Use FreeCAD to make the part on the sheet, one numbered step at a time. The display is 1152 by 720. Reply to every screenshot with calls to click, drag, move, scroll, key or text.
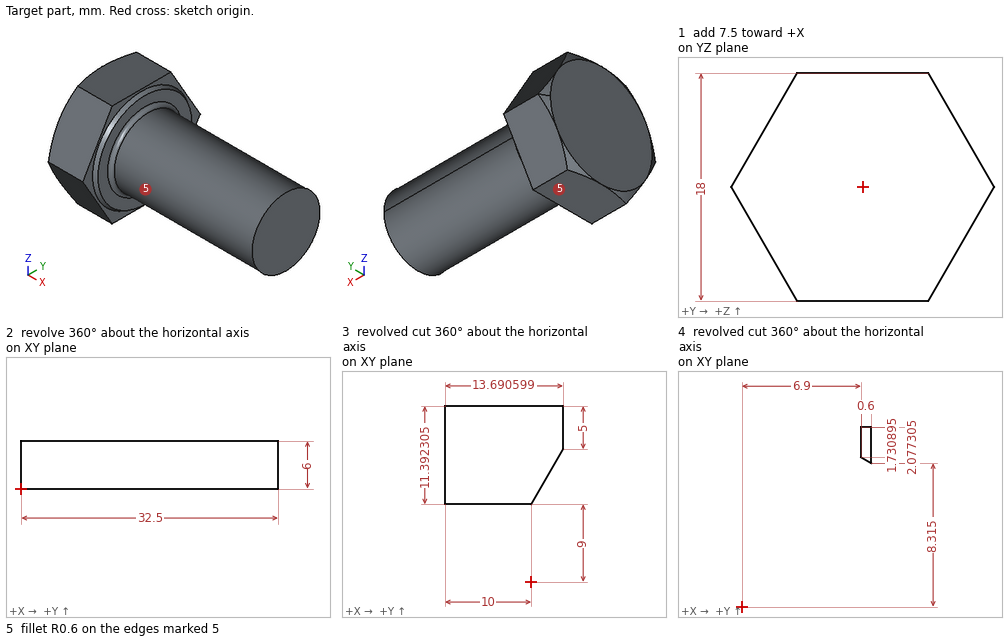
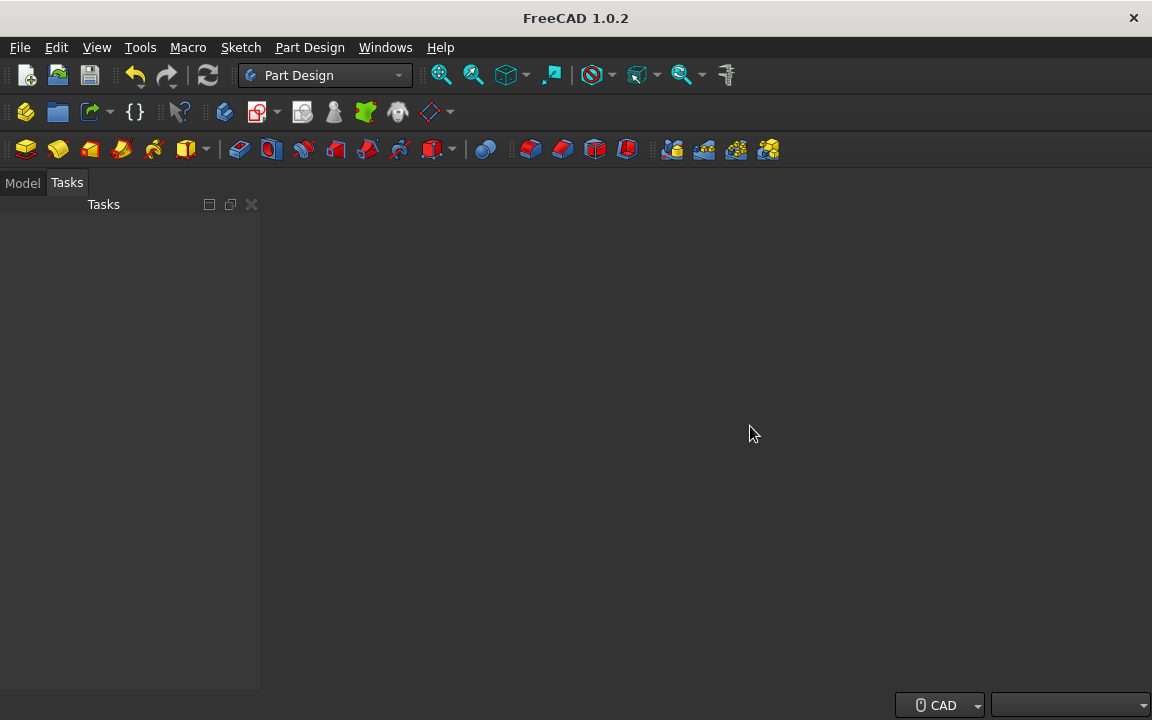
click(26, 76)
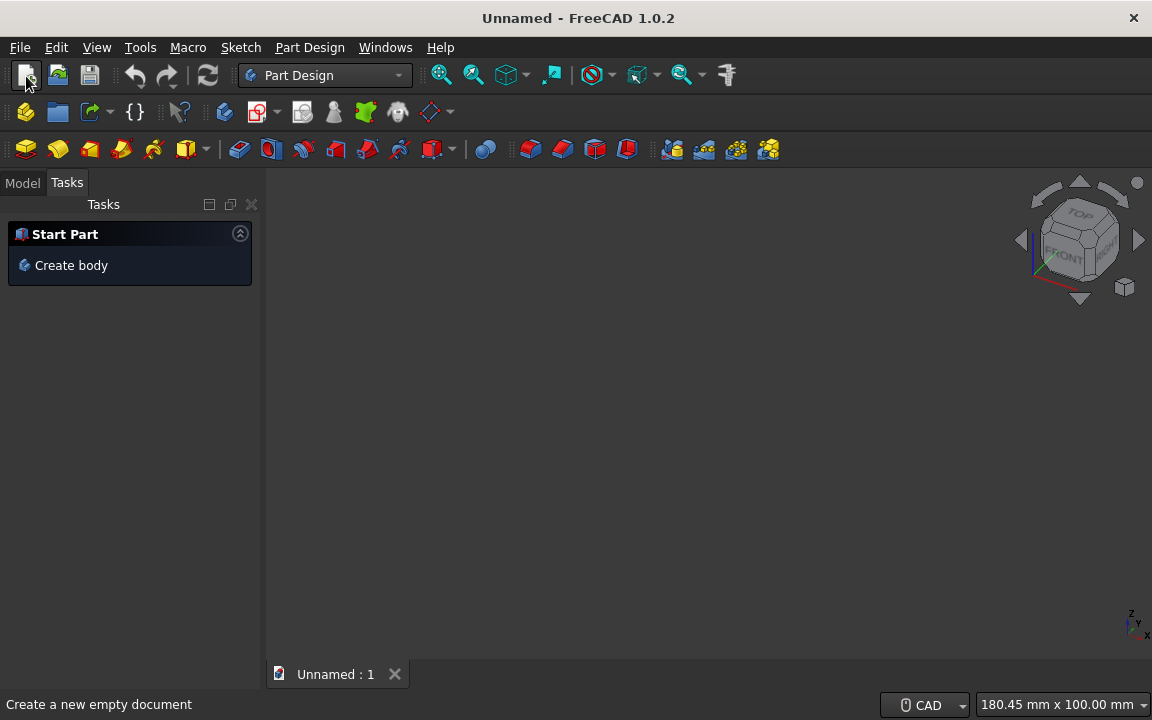
click(258, 112)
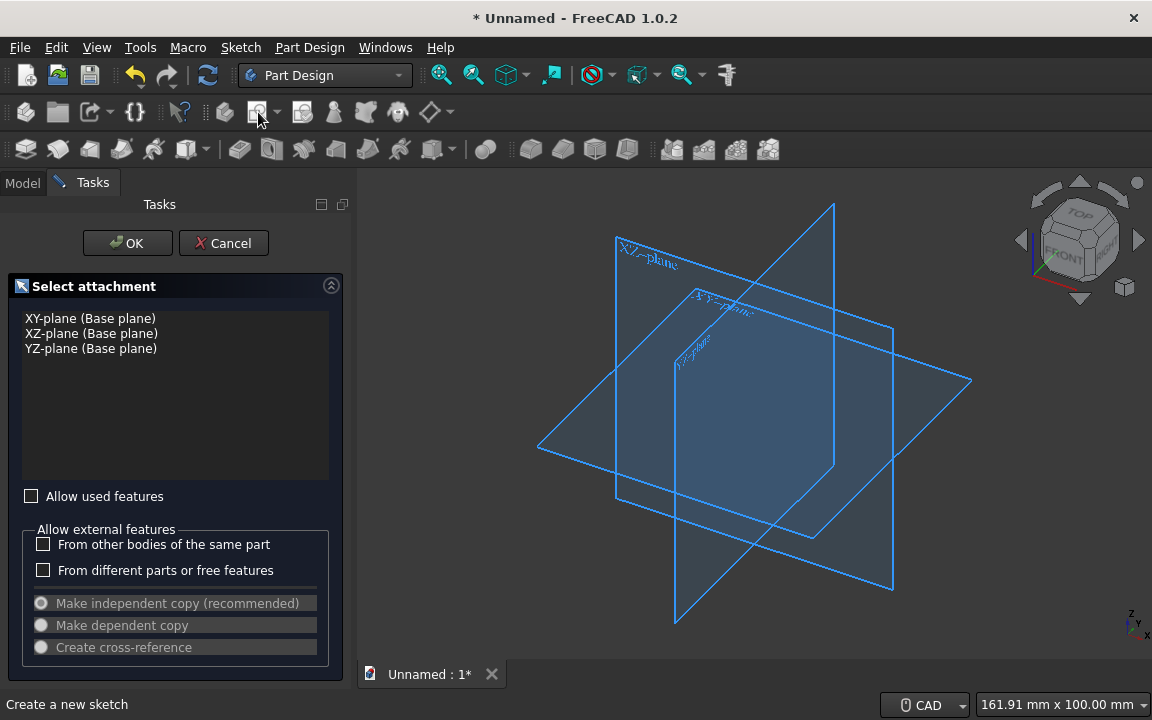
click(82, 348)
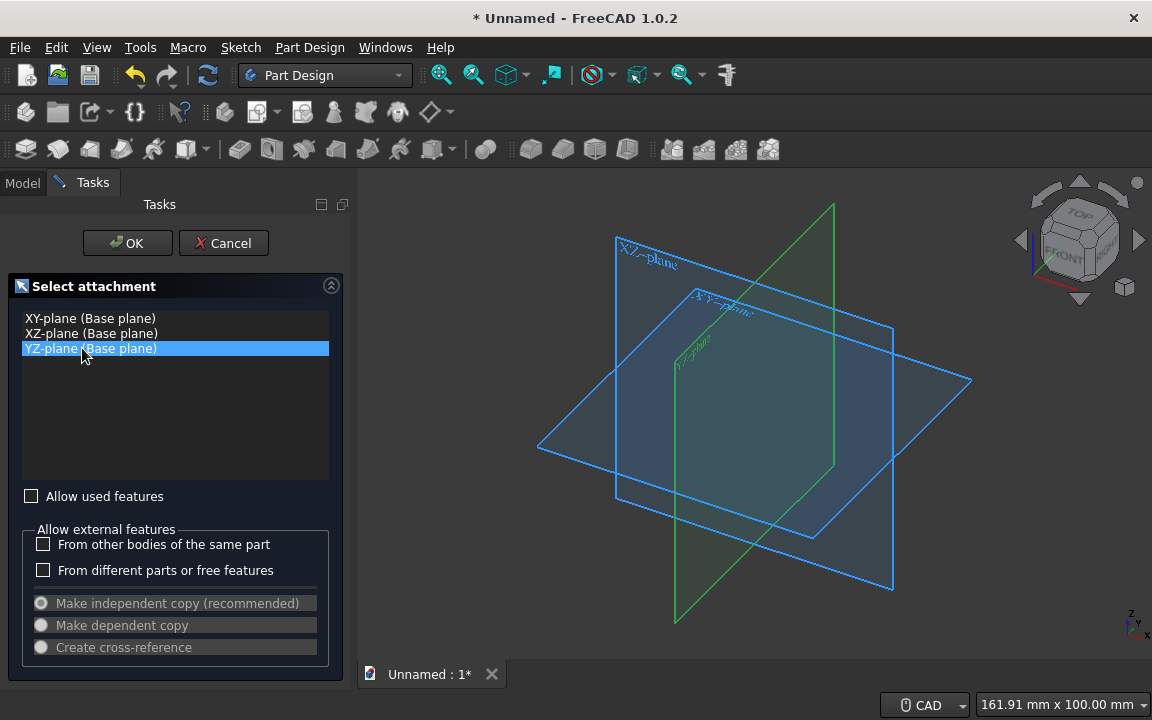
click(128, 243)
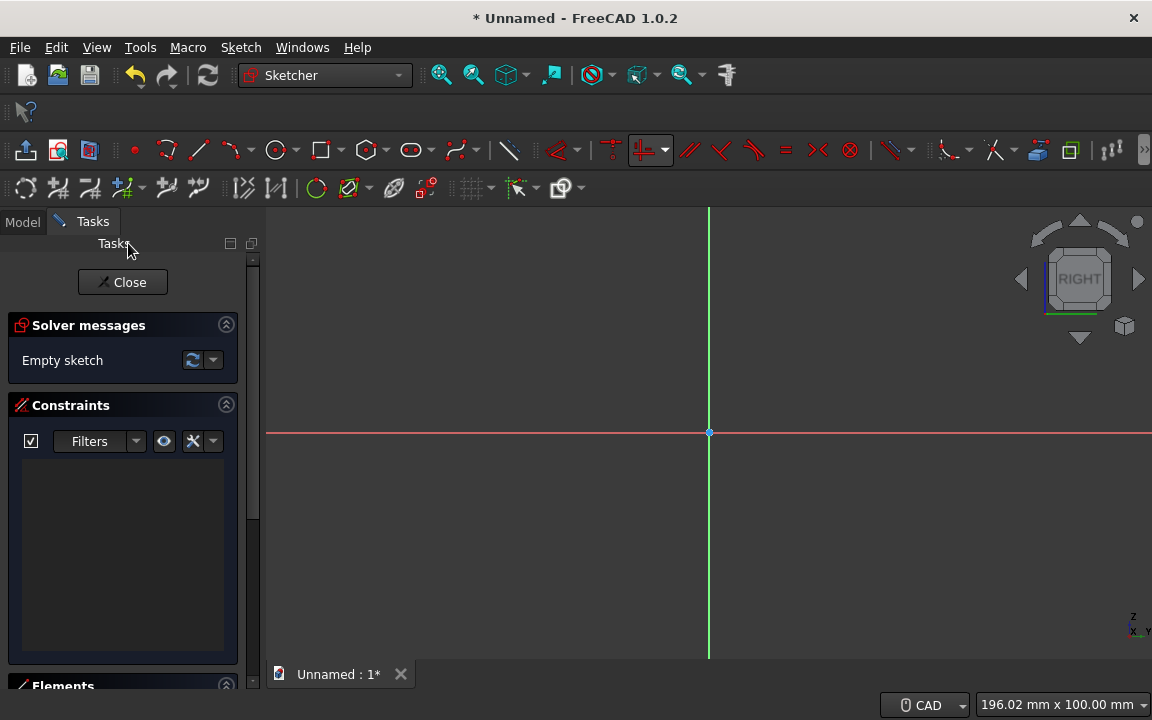
scroll(739, 433, up, 6)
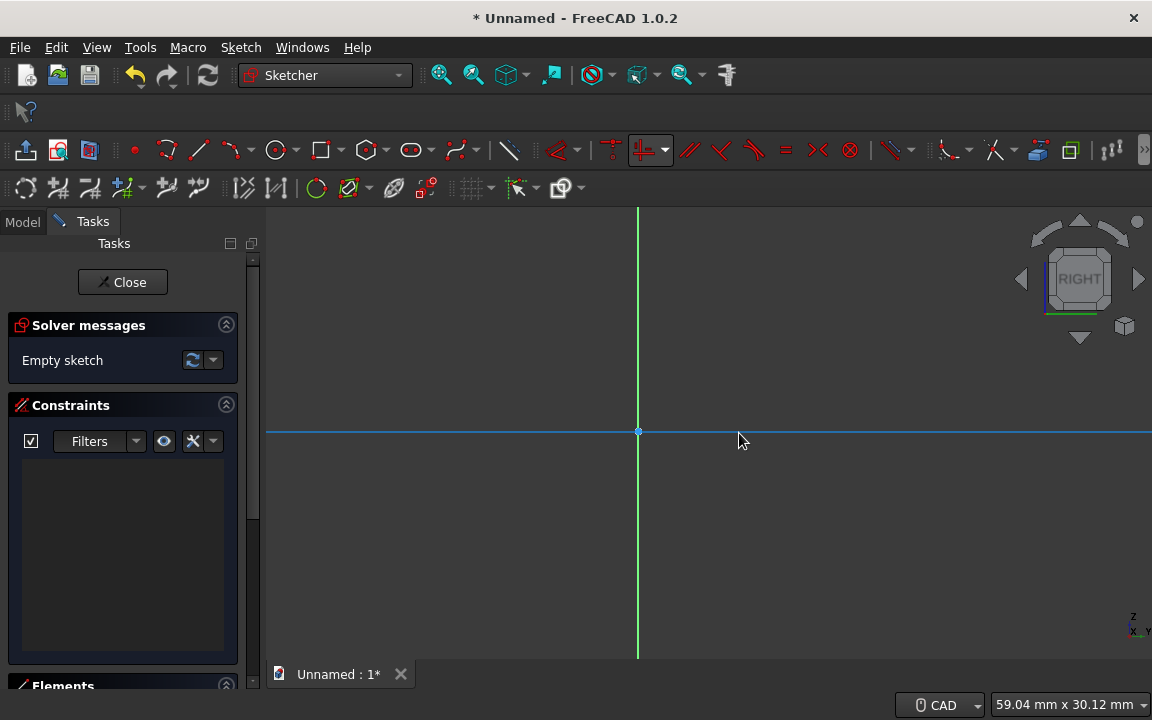
click(366, 150)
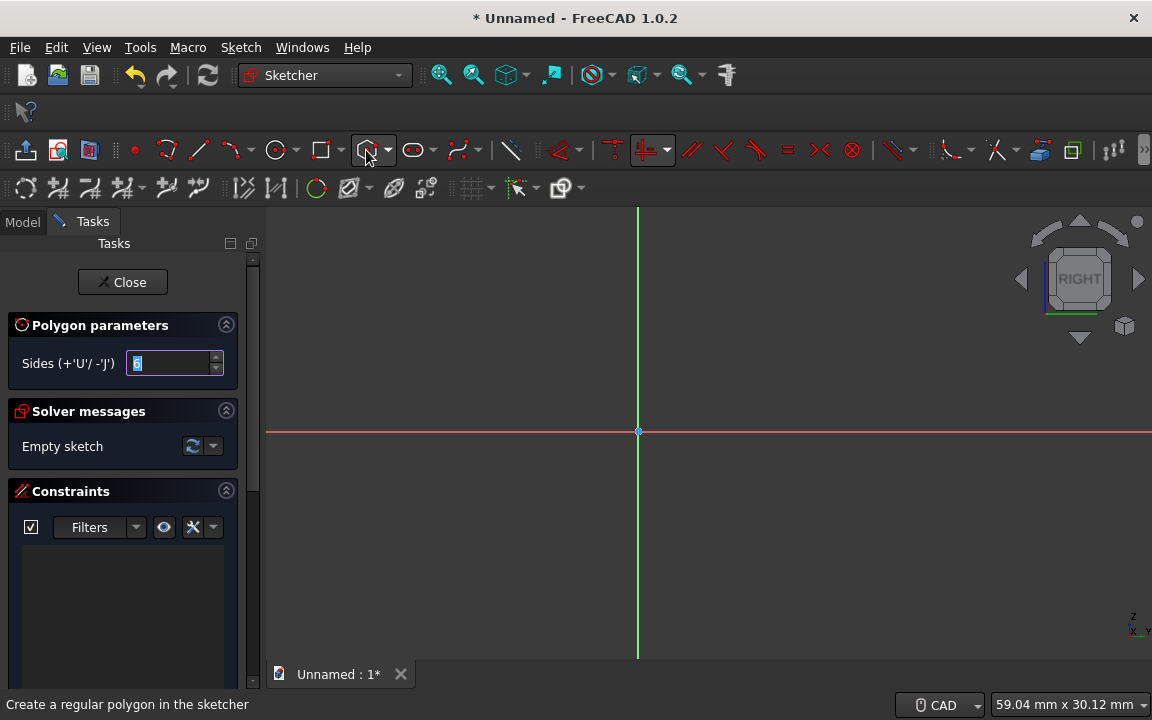
click(638, 432)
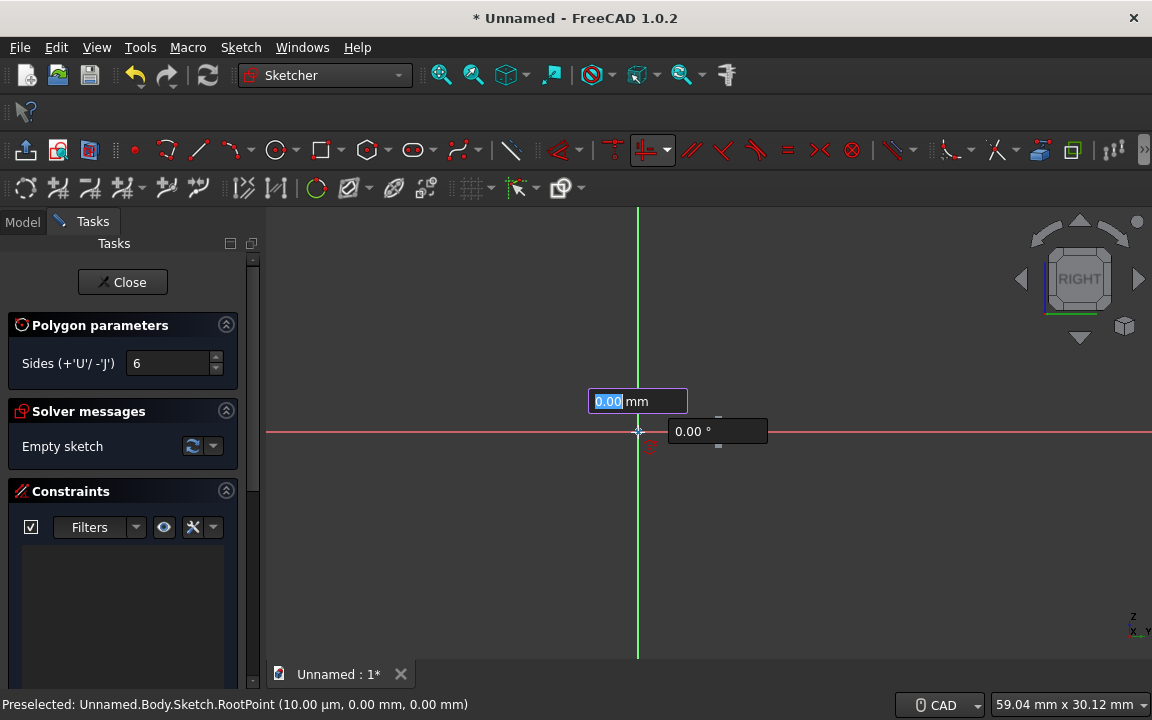
click(794, 432)
right_click(794, 432)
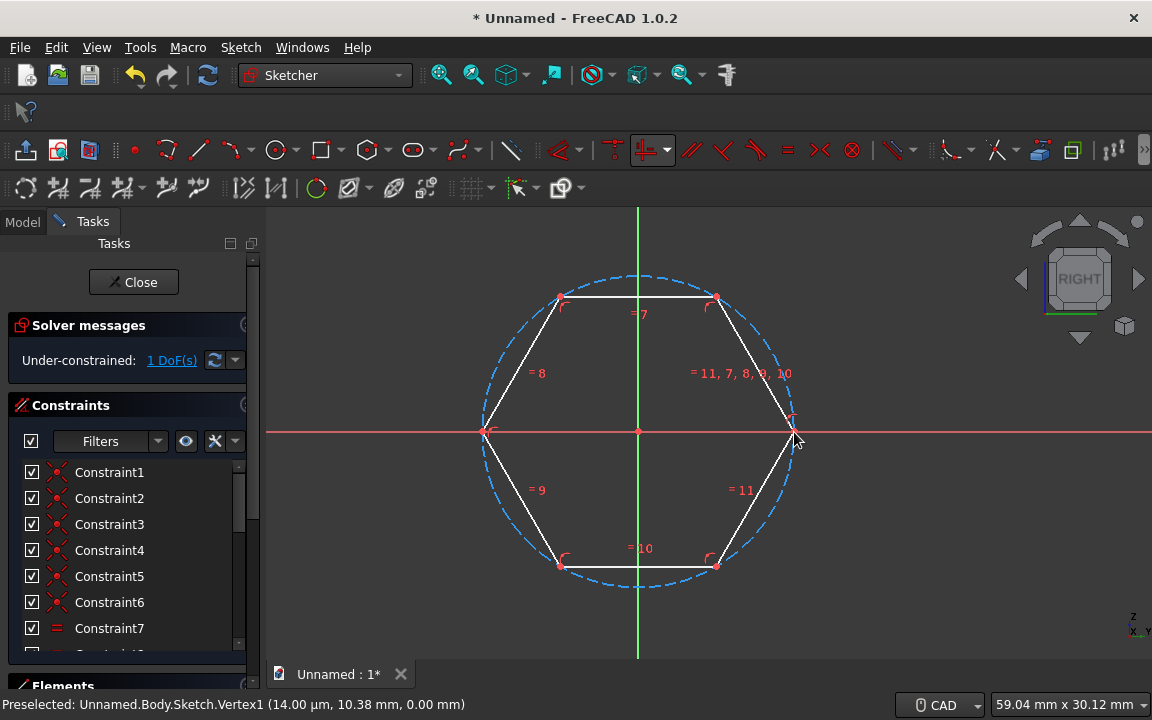
click(560, 567)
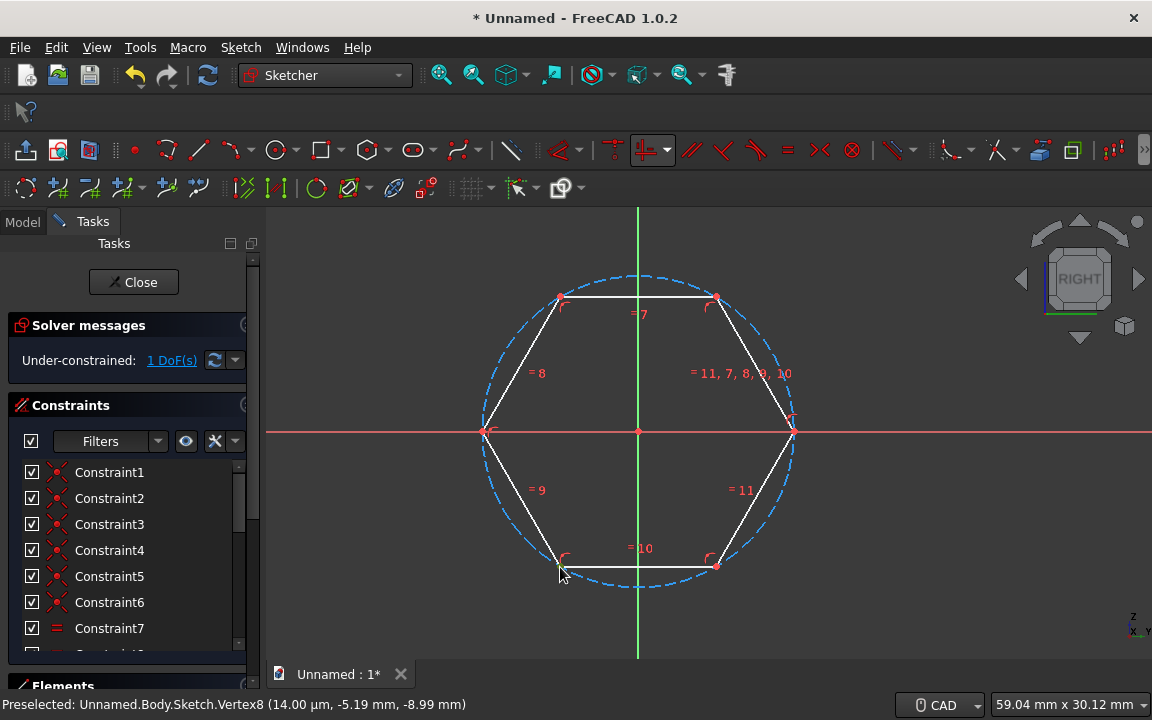
click(716, 297)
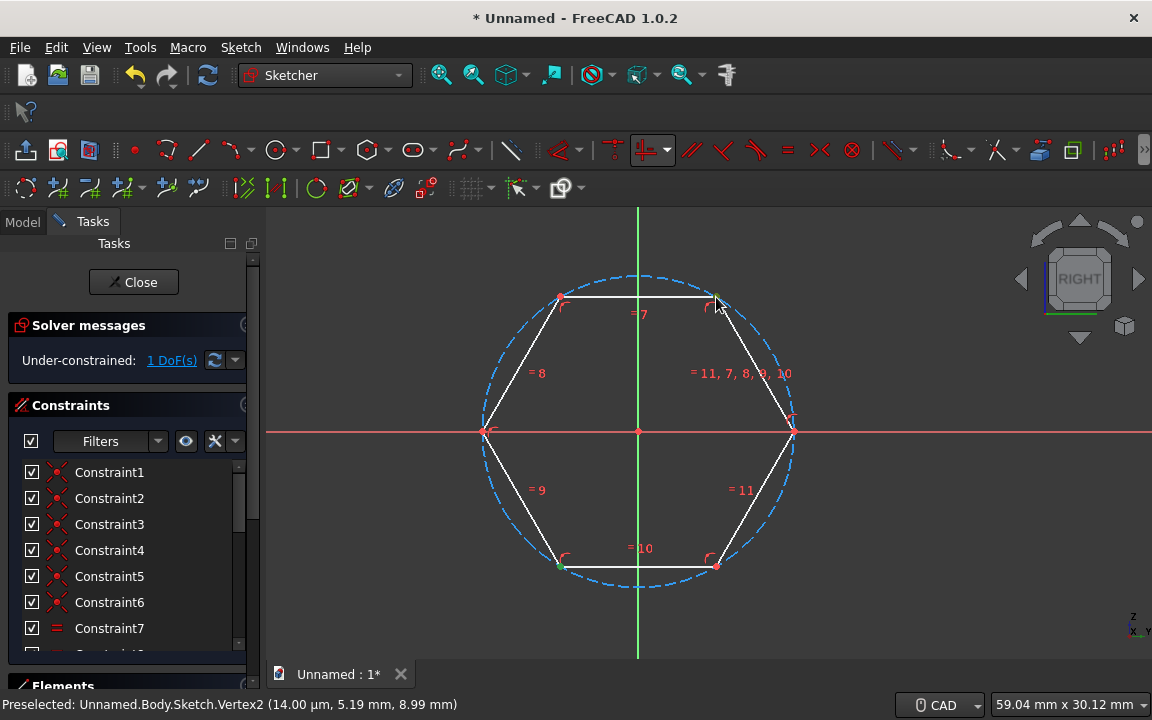
key(i)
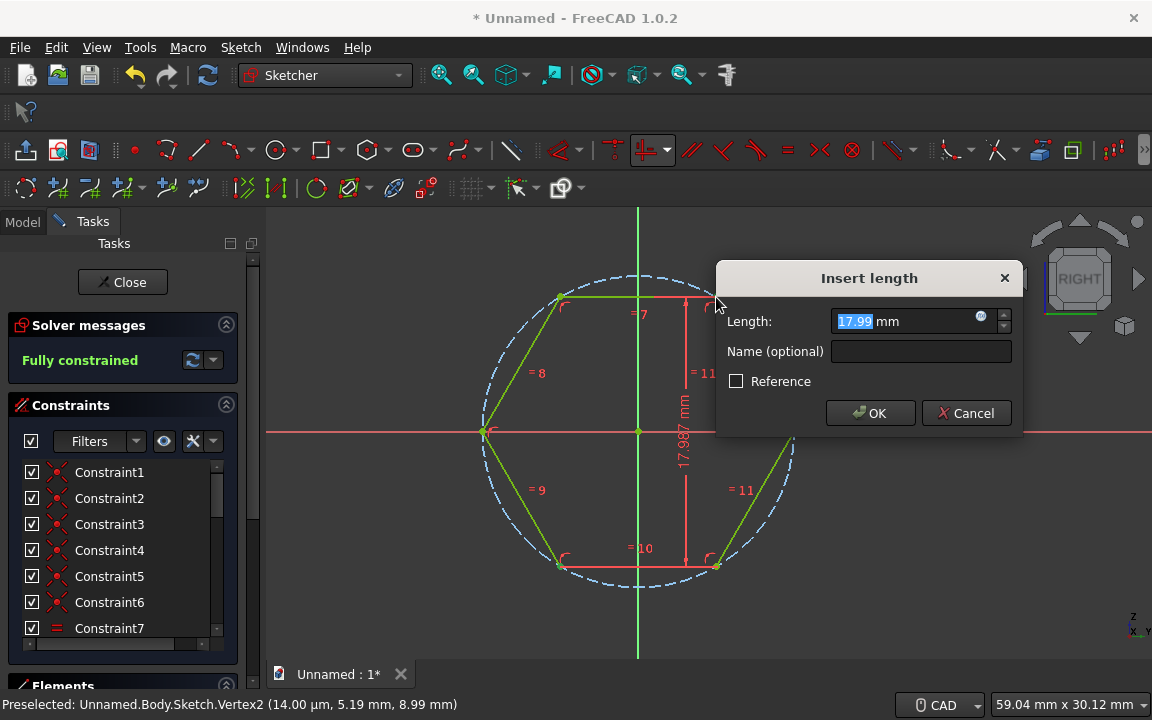
text(18)
key(Return)